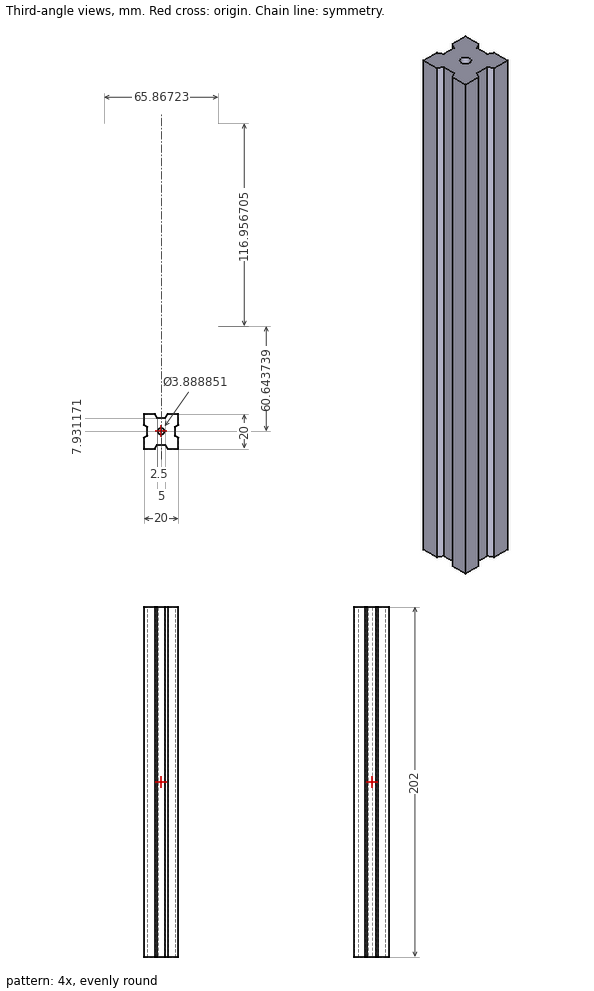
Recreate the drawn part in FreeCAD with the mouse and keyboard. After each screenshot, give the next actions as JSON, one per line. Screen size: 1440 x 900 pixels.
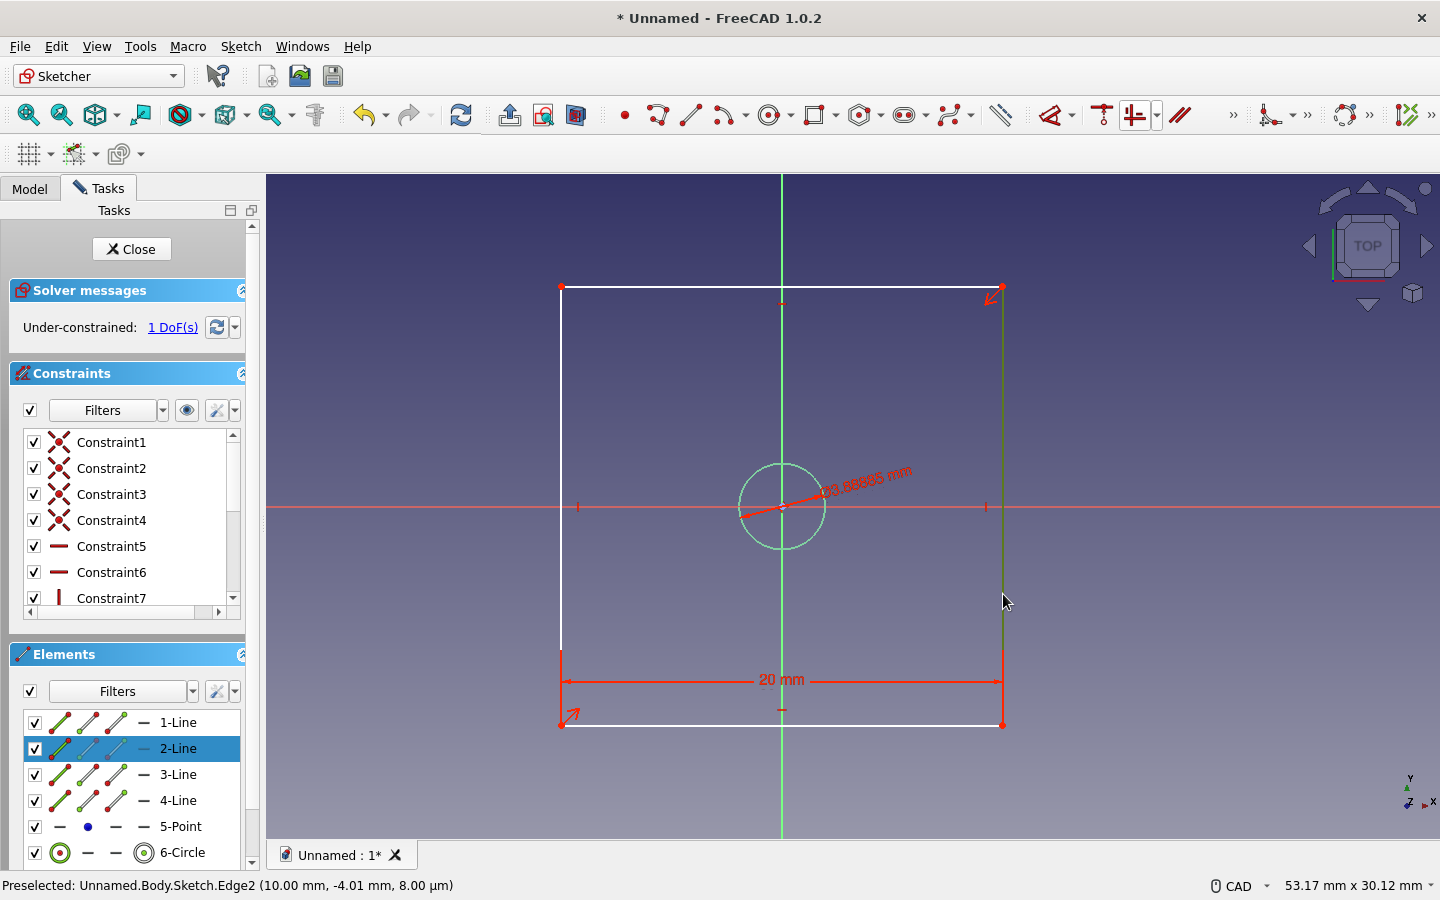
{"action": "key", "text": "i"}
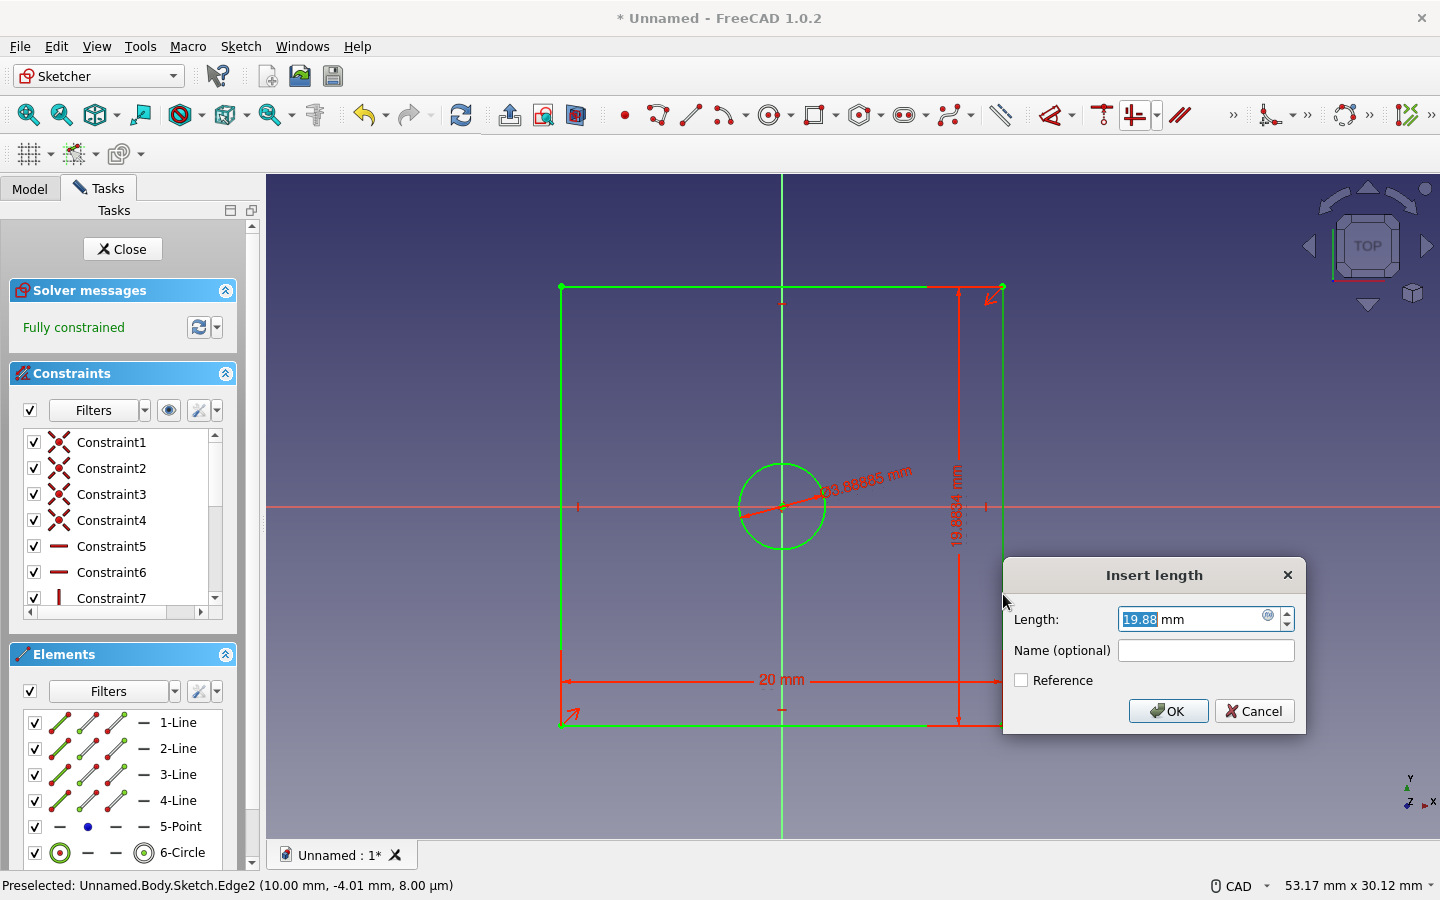
{"action": "type", "text": "20"}
{"action": "key", "text": "Return"}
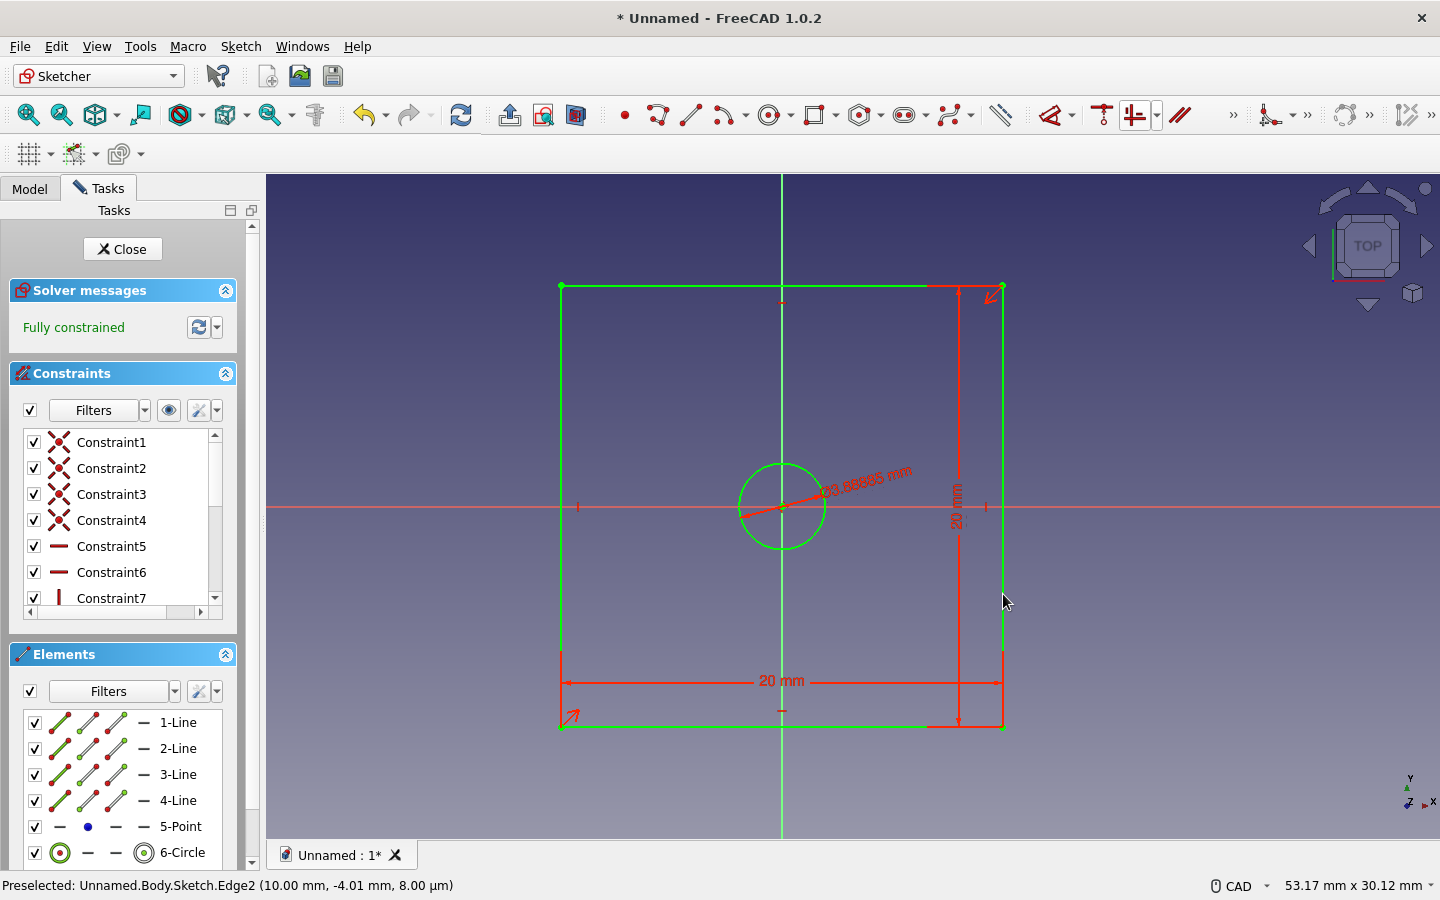
{"action": "left_click", "coordinate": [123, 249]}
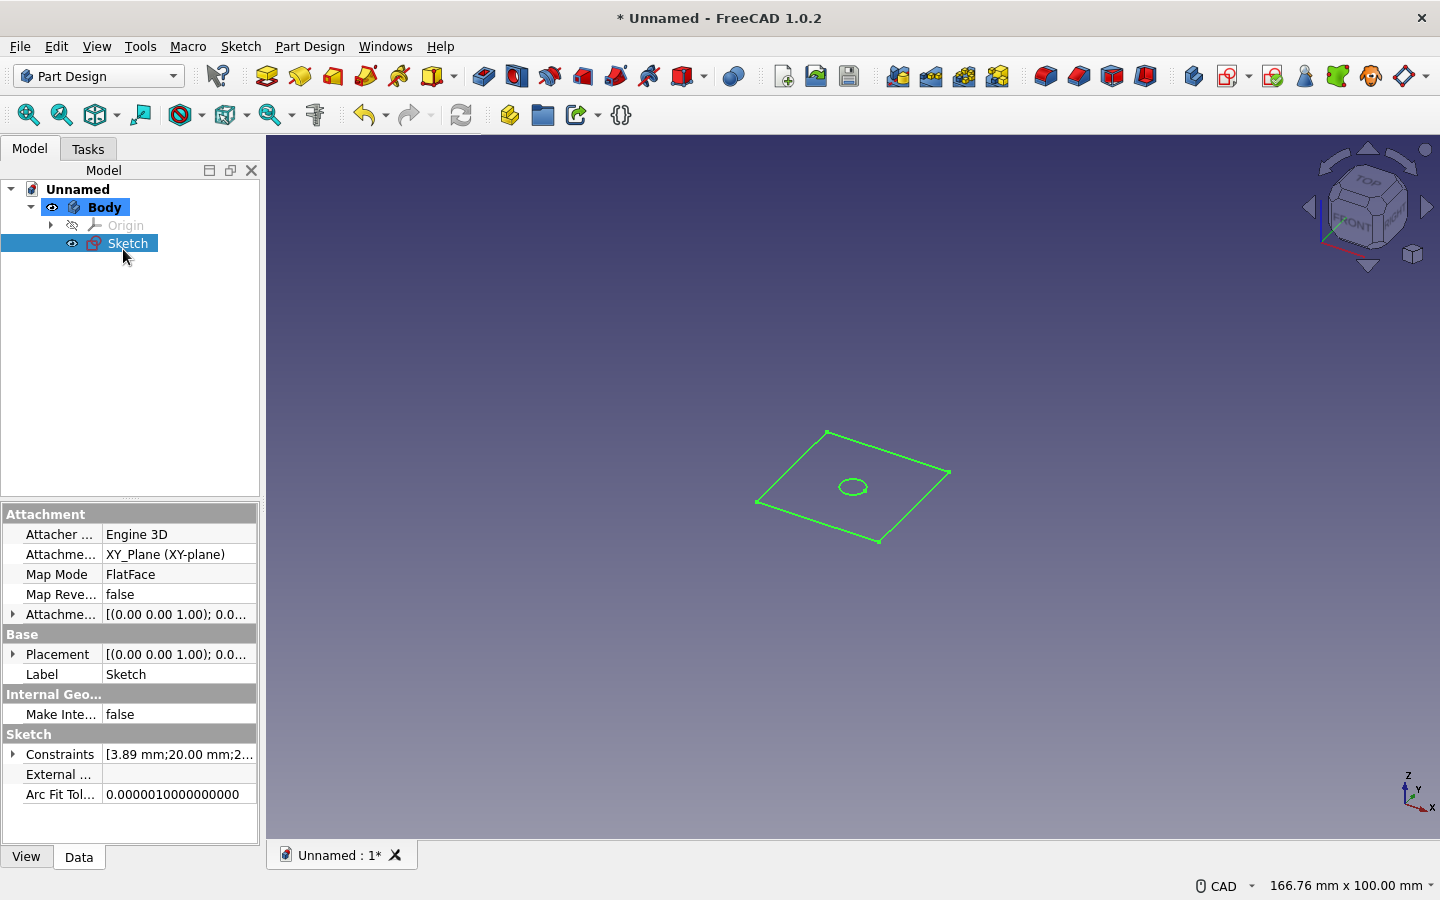
{"action": "left_click", "coordinate": [267, 76]}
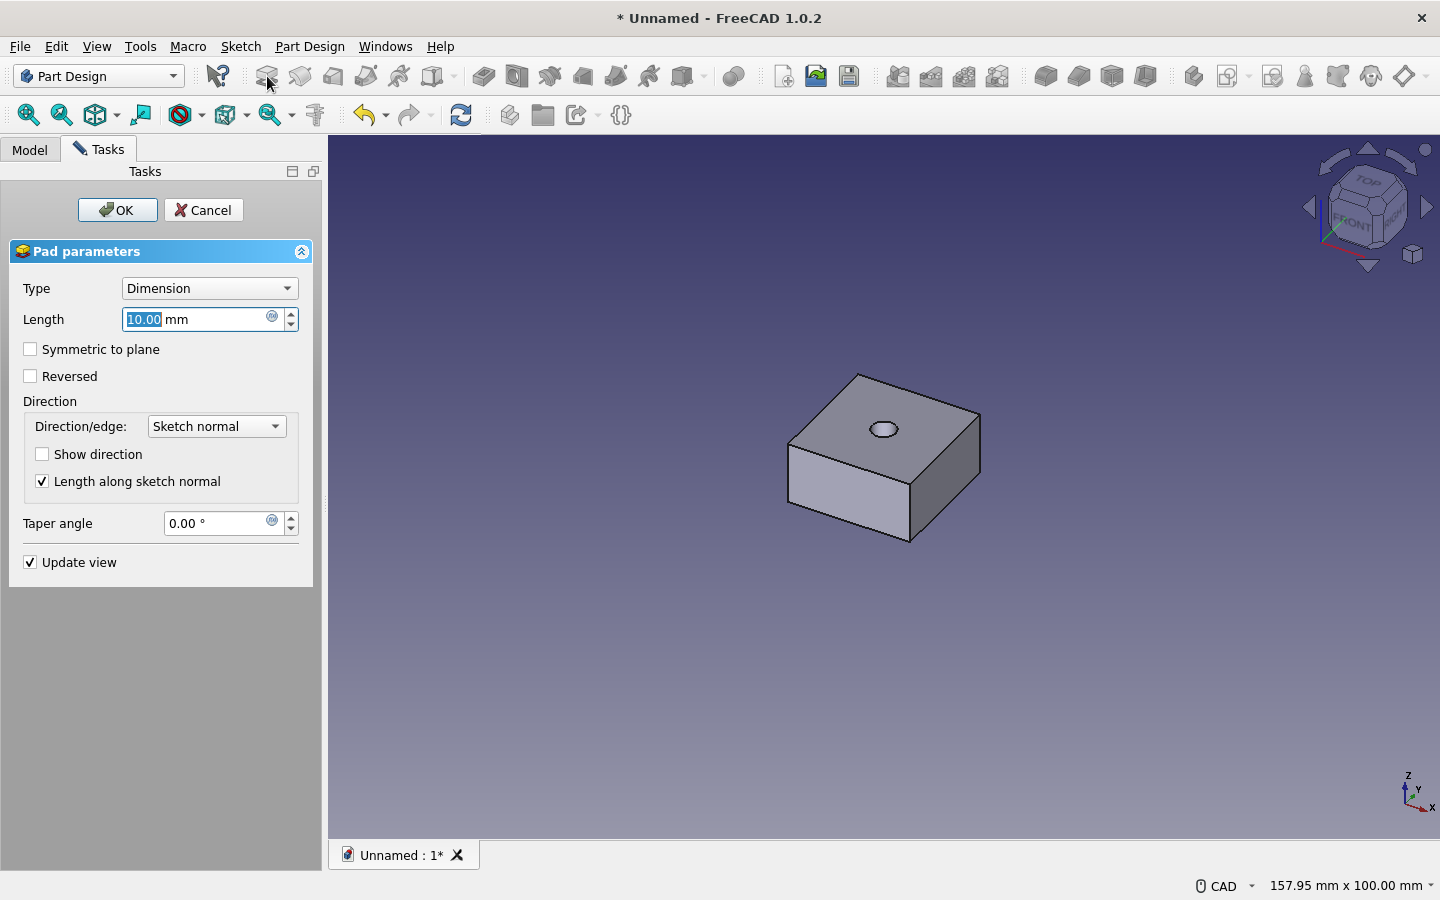
{"action": "type", "text": "202"}
{"action": "key", "text": "Tab"}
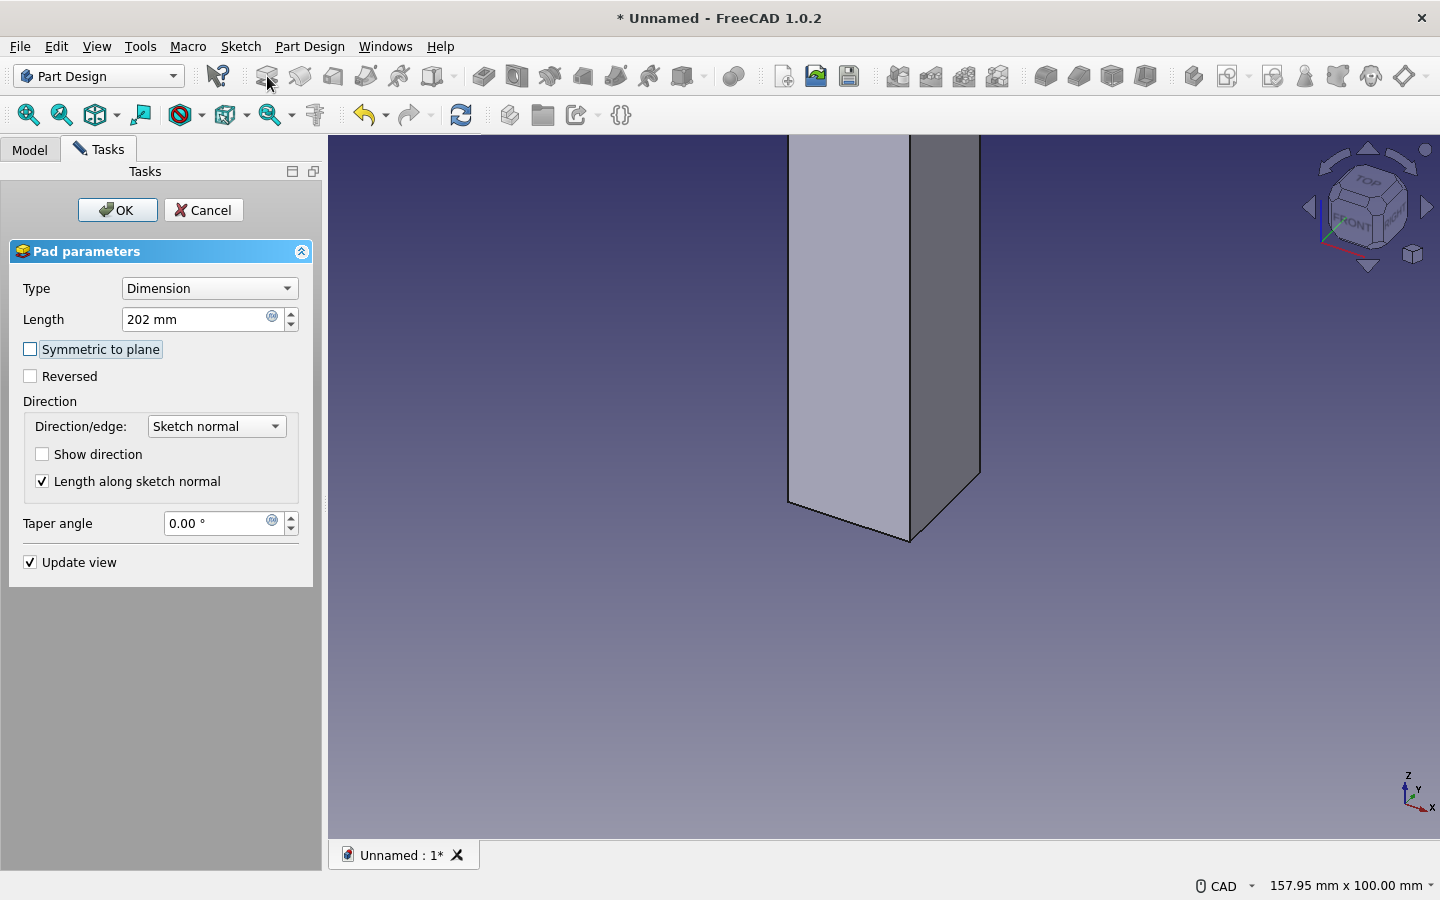
{"action": "left_click", "coordinate": [31, 349]}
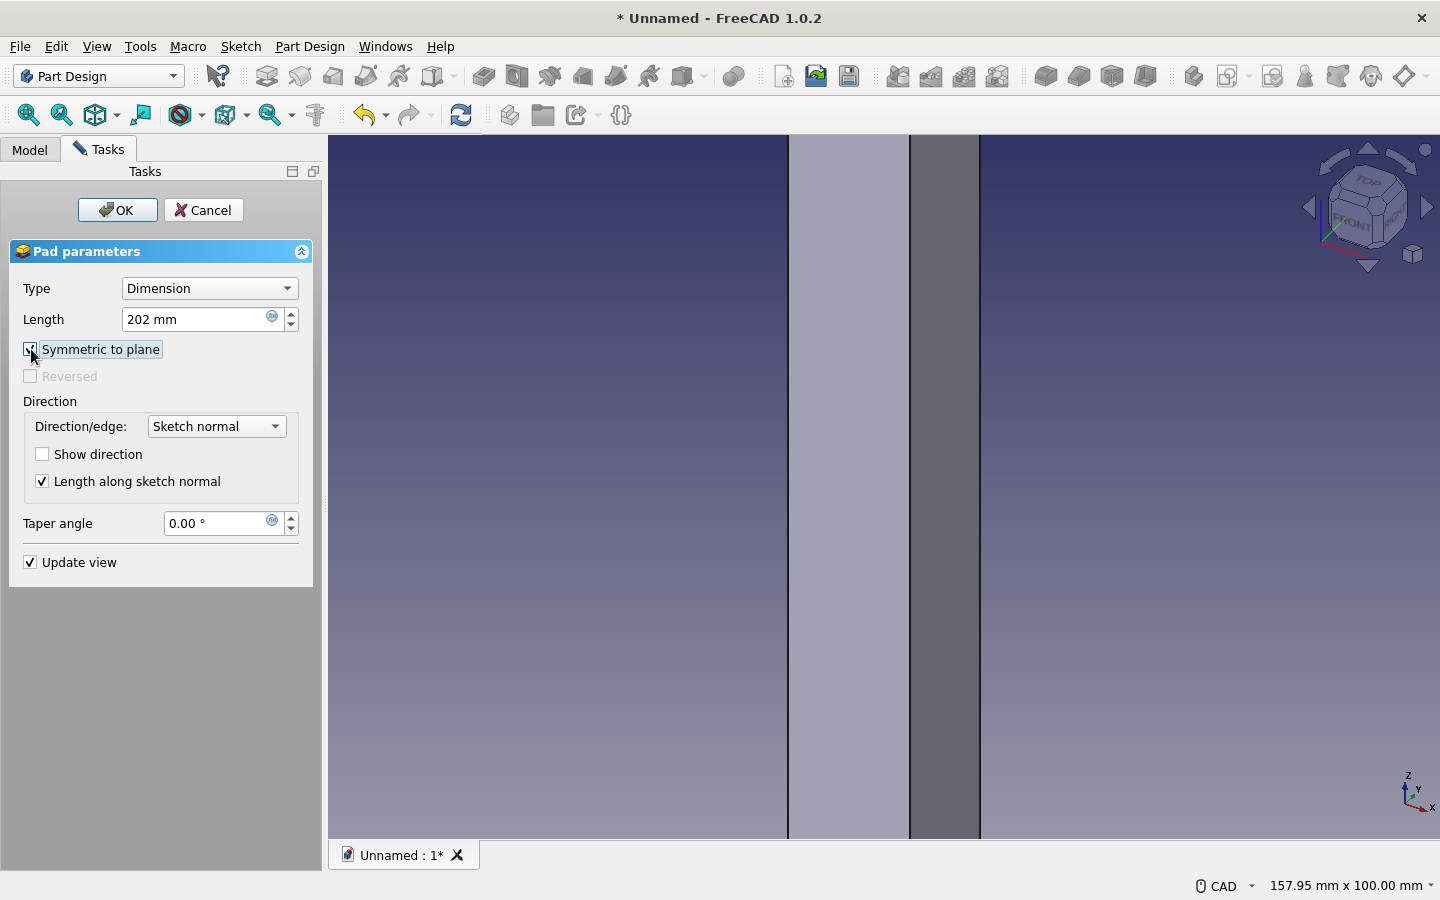
{"action": "left_click", "coordinate": [118, 210]}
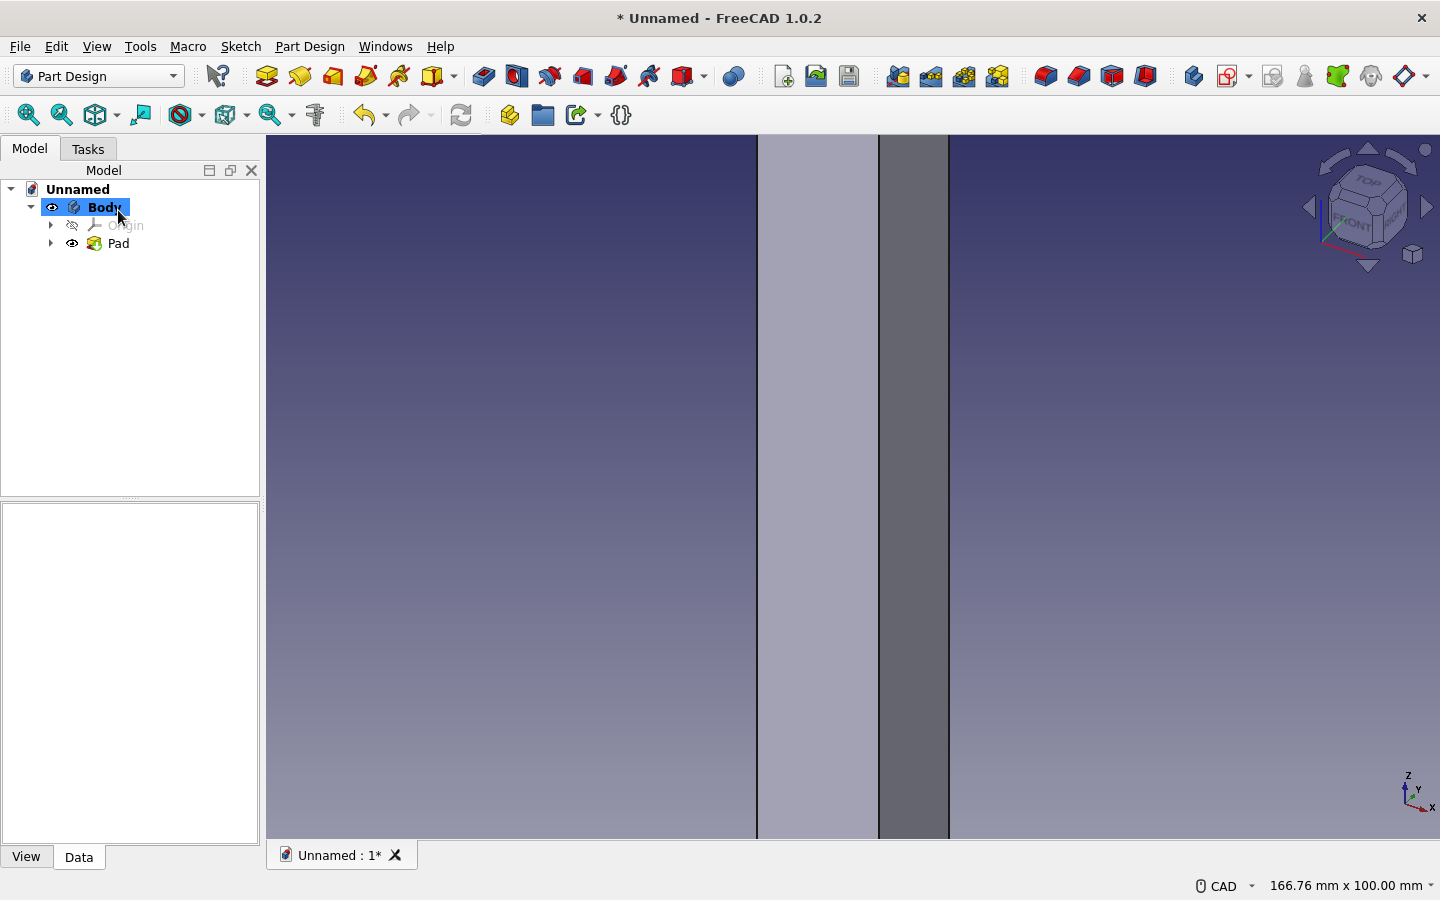
{"action": "key", "text": "v f"}